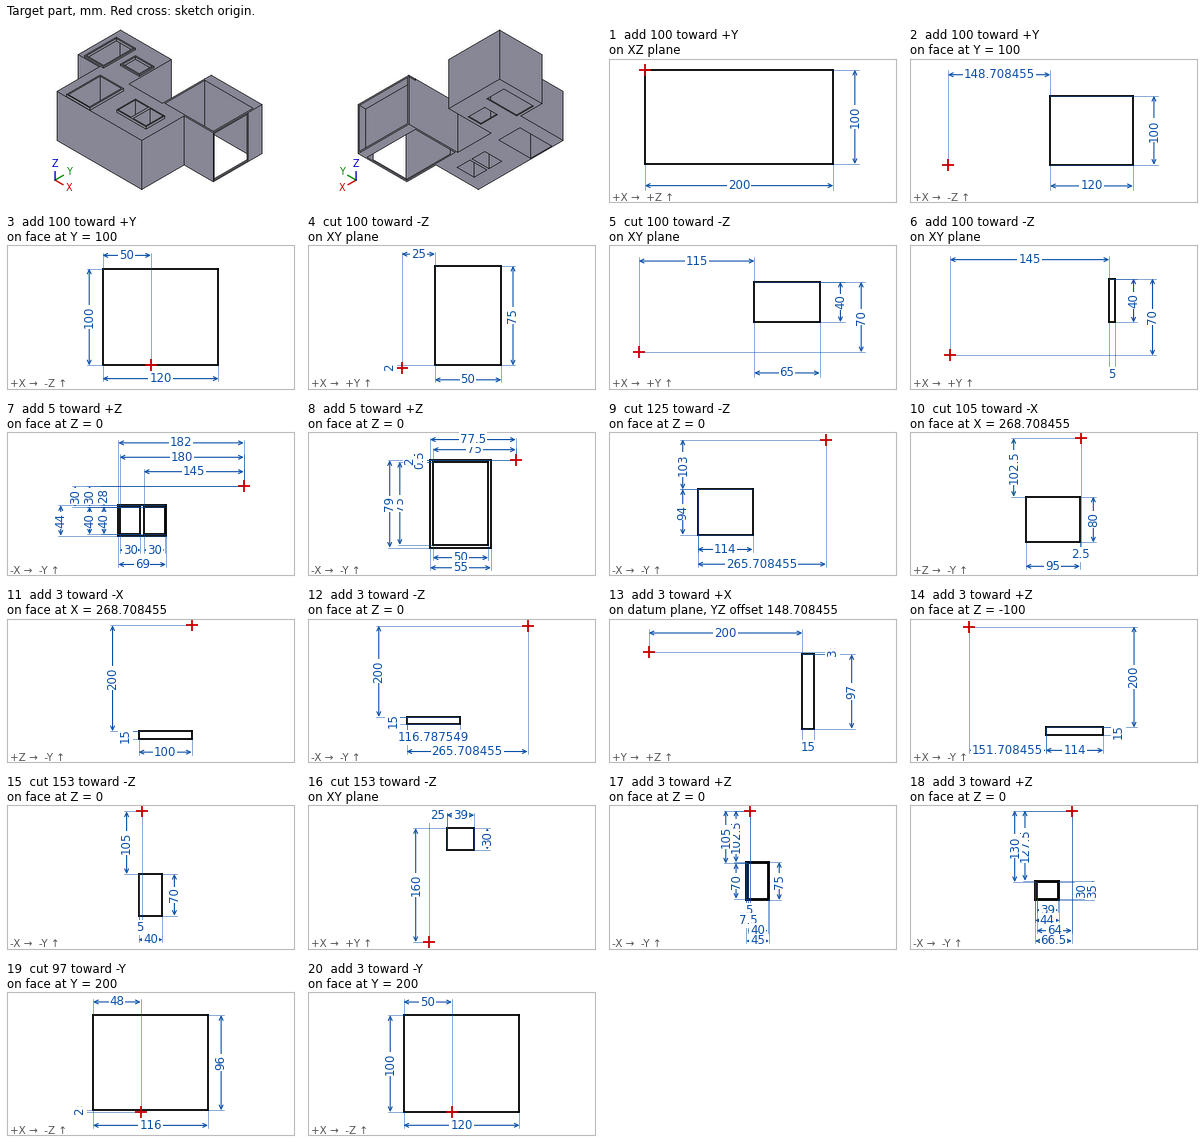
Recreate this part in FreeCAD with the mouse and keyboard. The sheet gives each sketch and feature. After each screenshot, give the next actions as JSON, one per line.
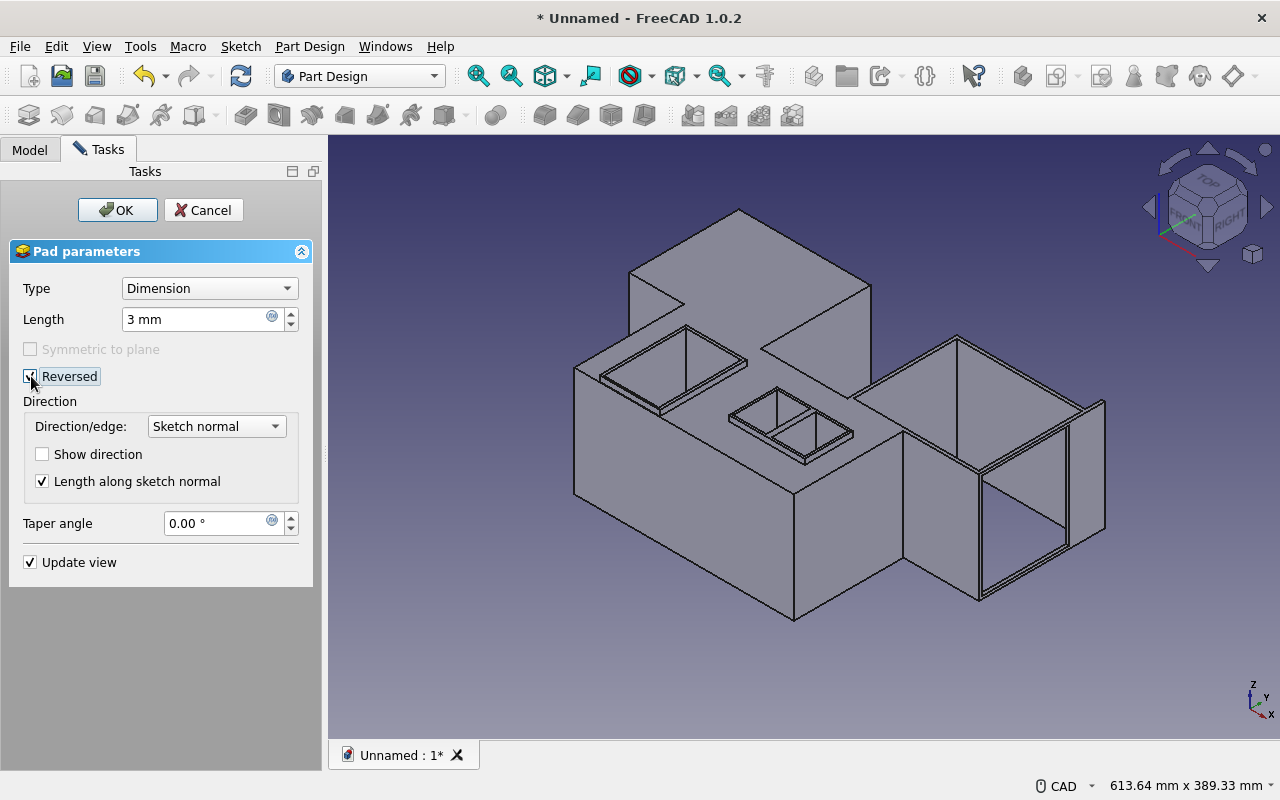
{"action": "left_click", "coordinate": [118, 210]}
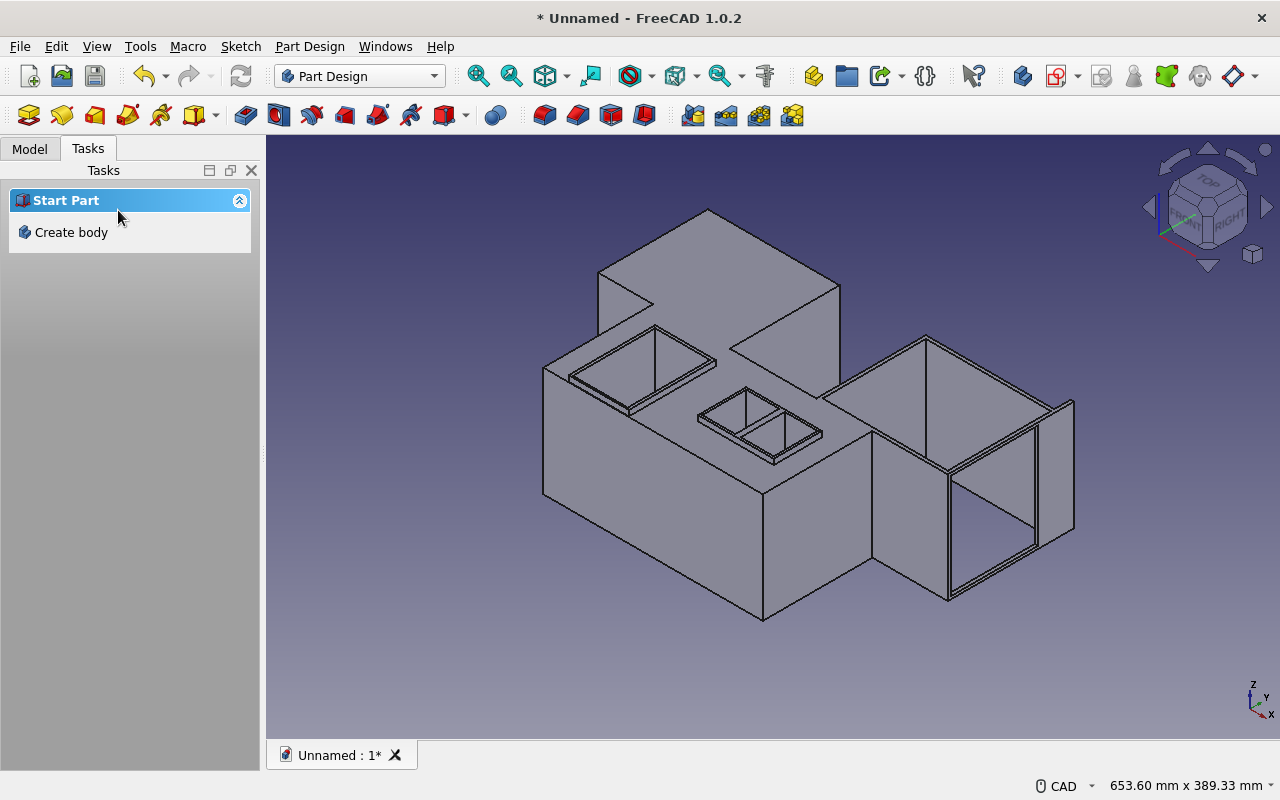
{"action": "left_click", "coordinate": [715, 291]}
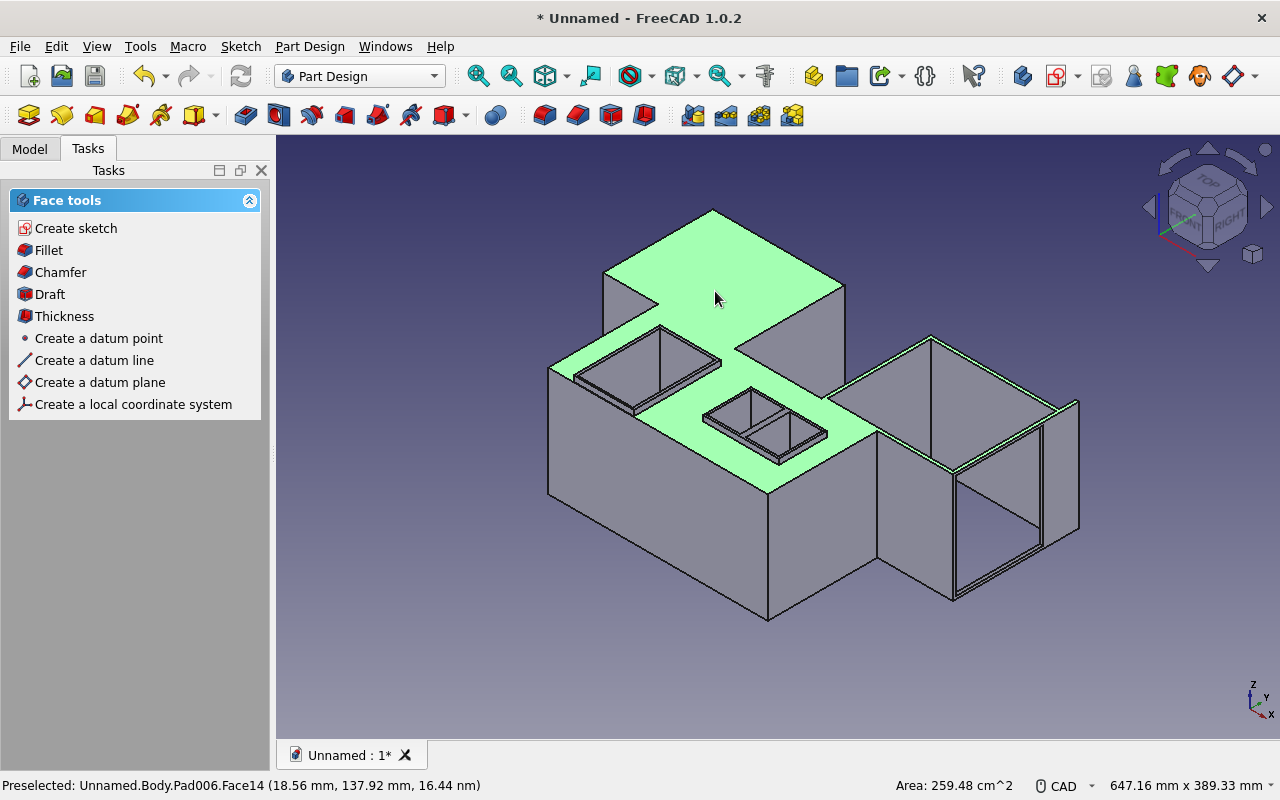
{"action": "left_click", "coordinate": [1056, 76]}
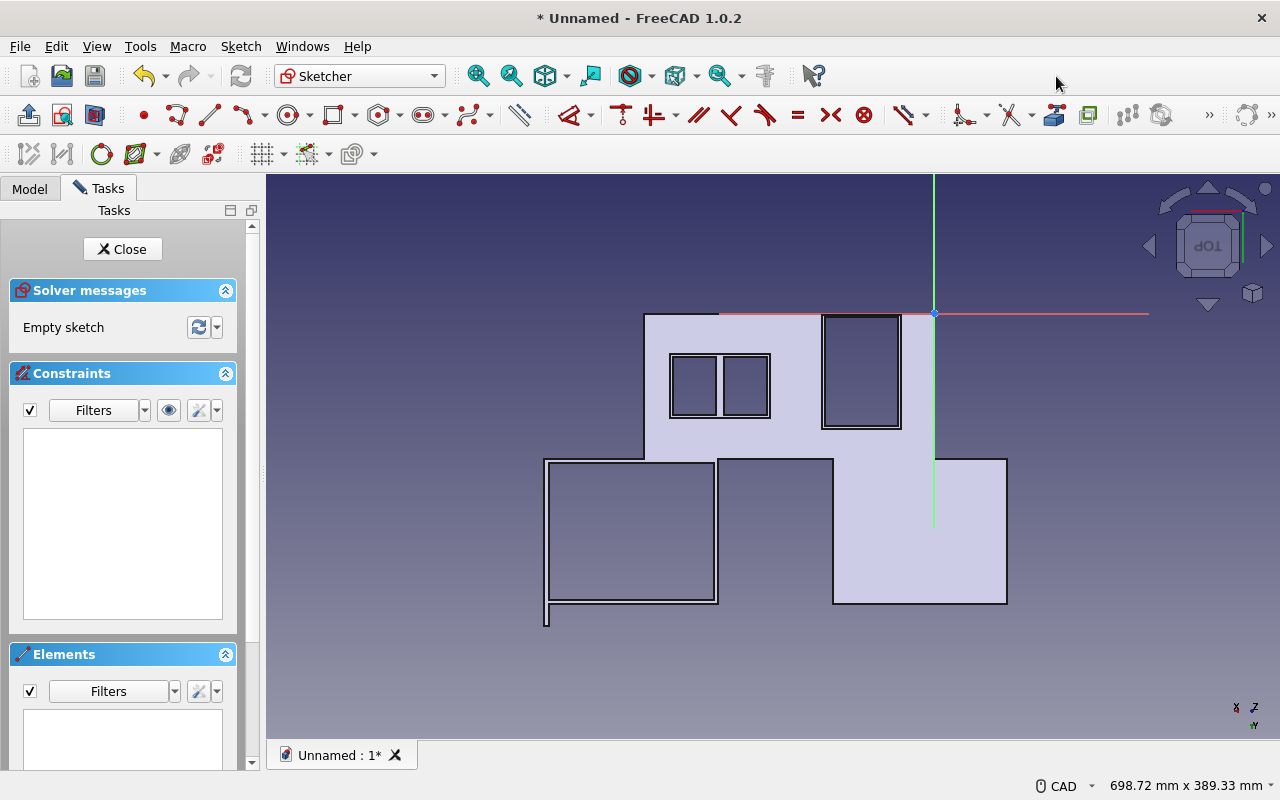
{"action": "left_click", "coordinate": [332, 116]}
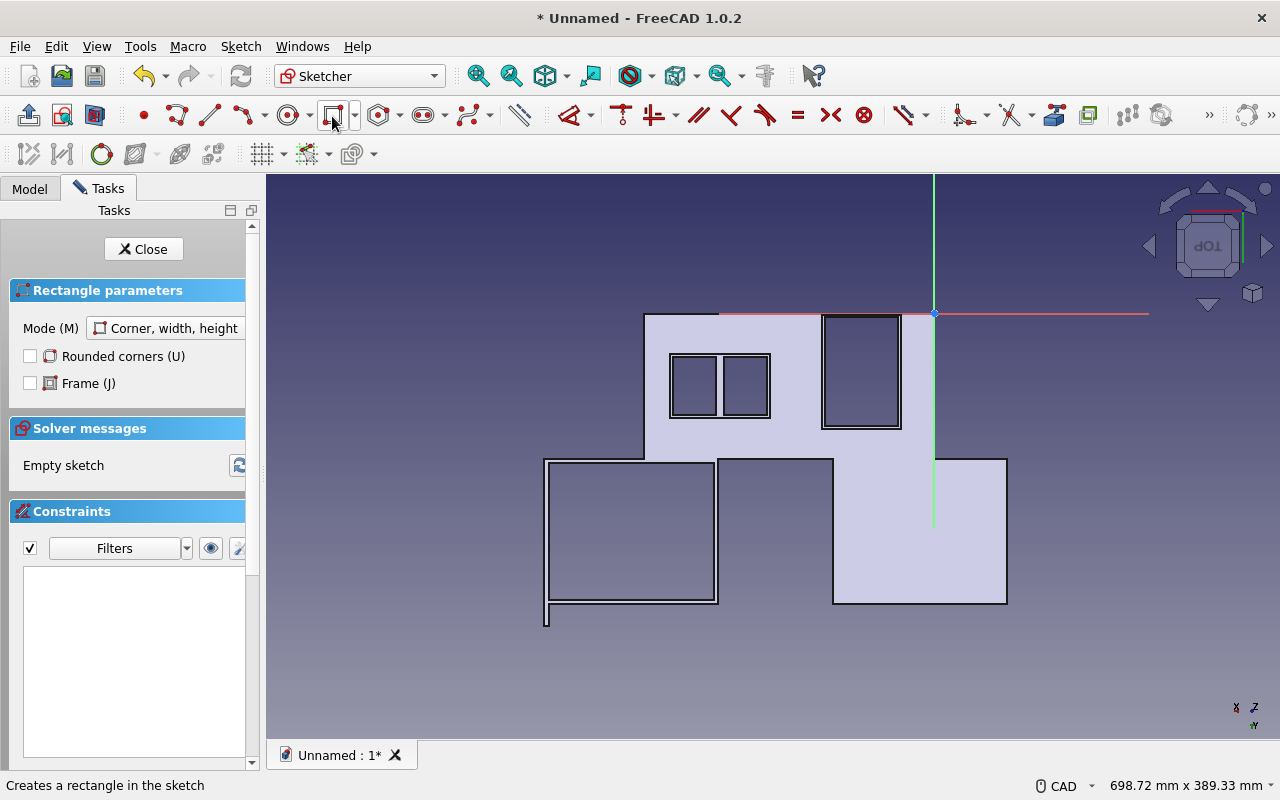
{"action": "left_click", "coordinate": [549, 604]}
{"action": "mouse_move", "coordinate": [718, 626]}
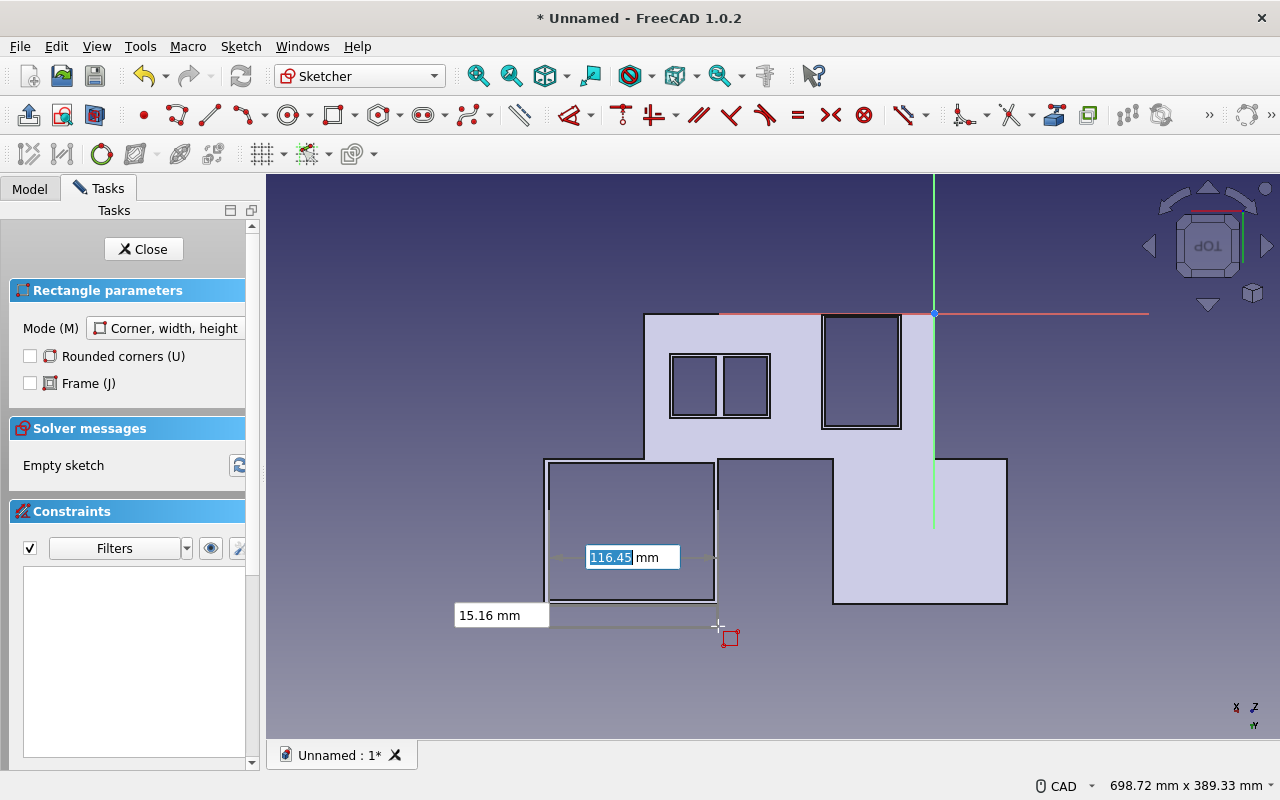
{"action": "type", "text": "116.787549"}
{"action": "key", "text": "Tab"}
{"action": "type", "text": "15"}
{"action": "key", "text": "Return"}
{"action": "key", "text": "Escape"}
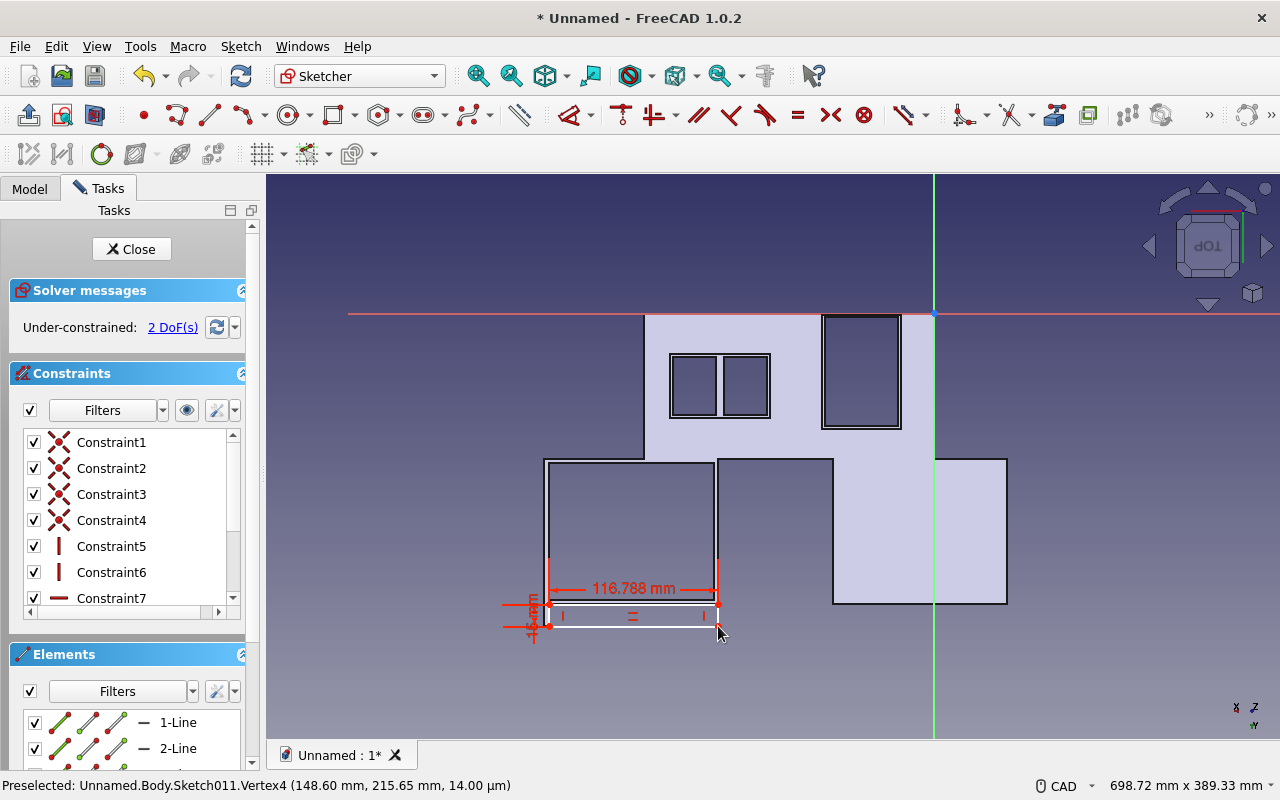
{"action": "left_click", "coordinate": [568, 116]}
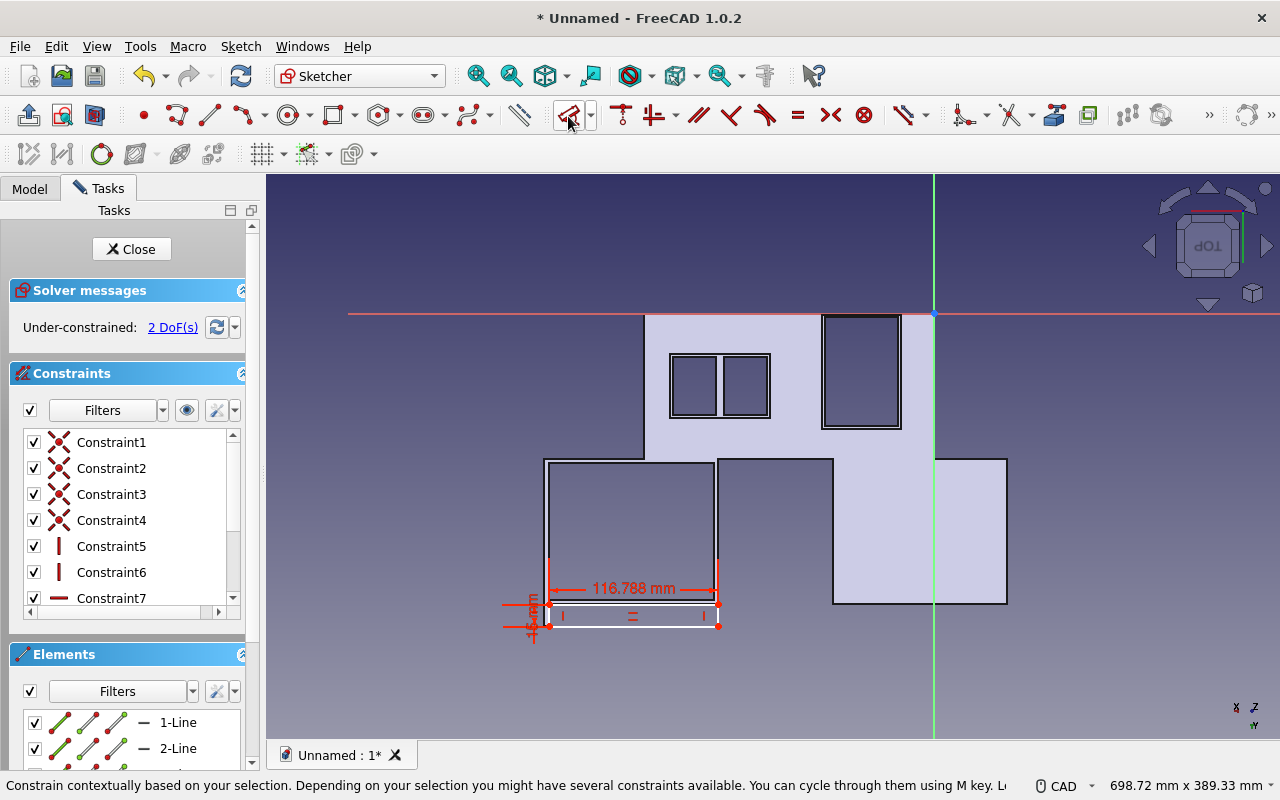
{"action": "left_click", "coordinate": [549, 605]}
{"action": "left_click", "coordinate": [968, 459]}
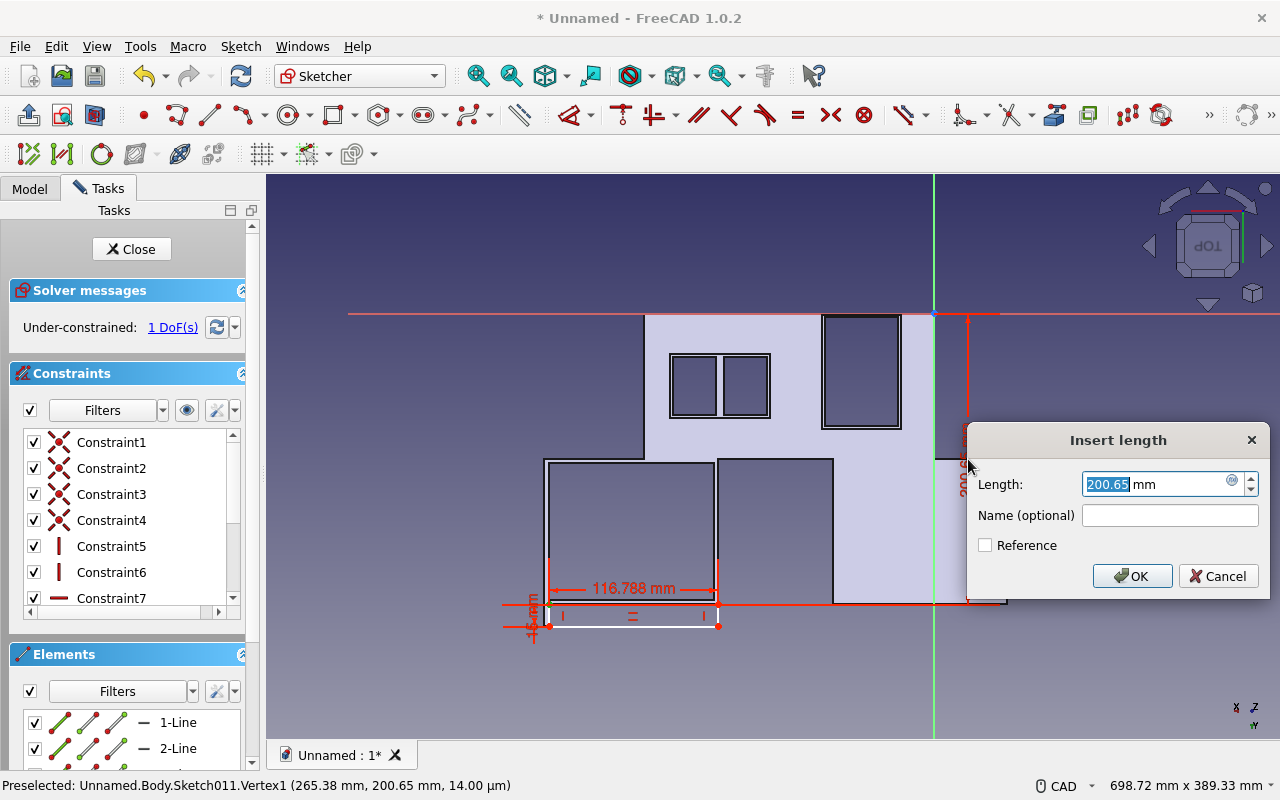
{"action": "type", "text": "200"}
{"action": "key", "text": "Return"}